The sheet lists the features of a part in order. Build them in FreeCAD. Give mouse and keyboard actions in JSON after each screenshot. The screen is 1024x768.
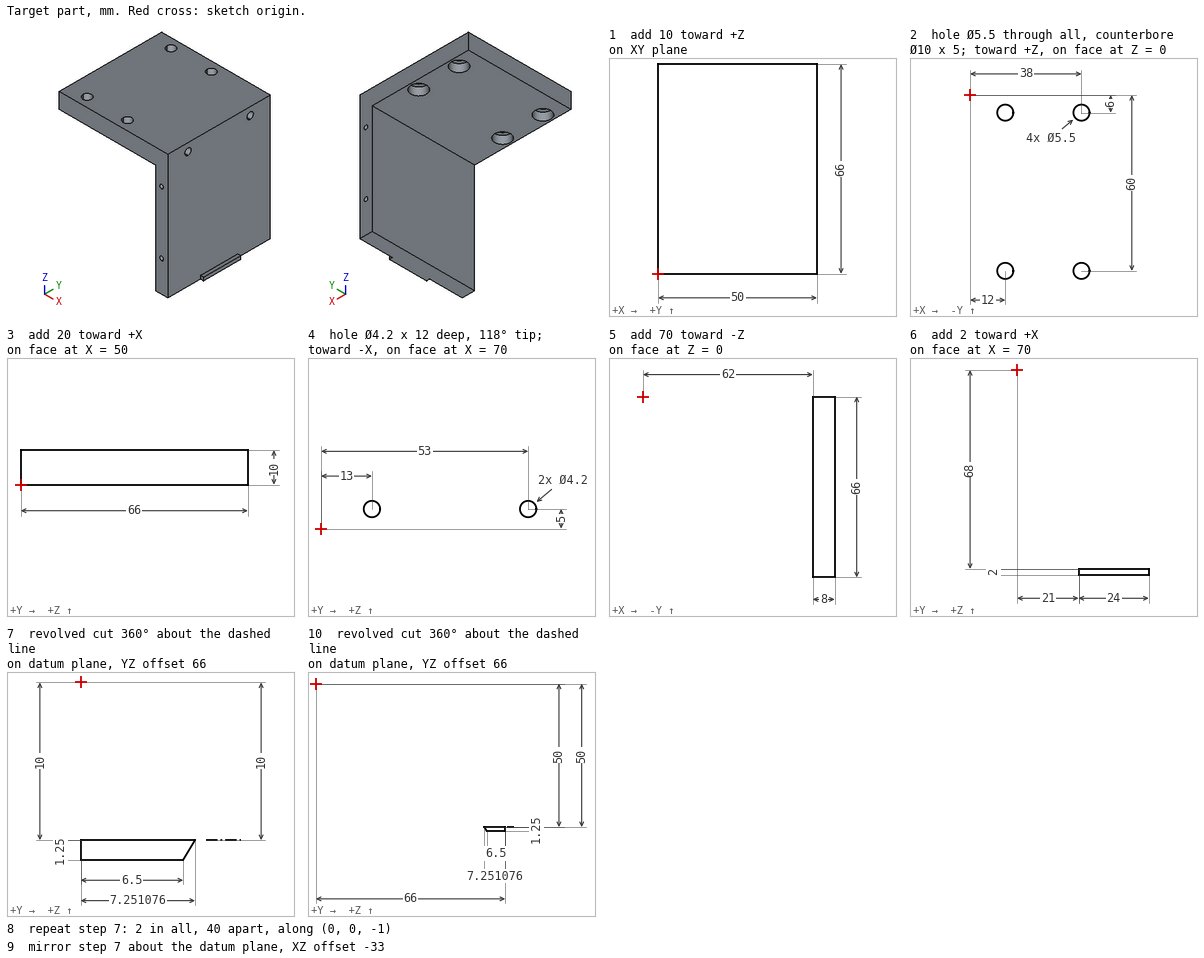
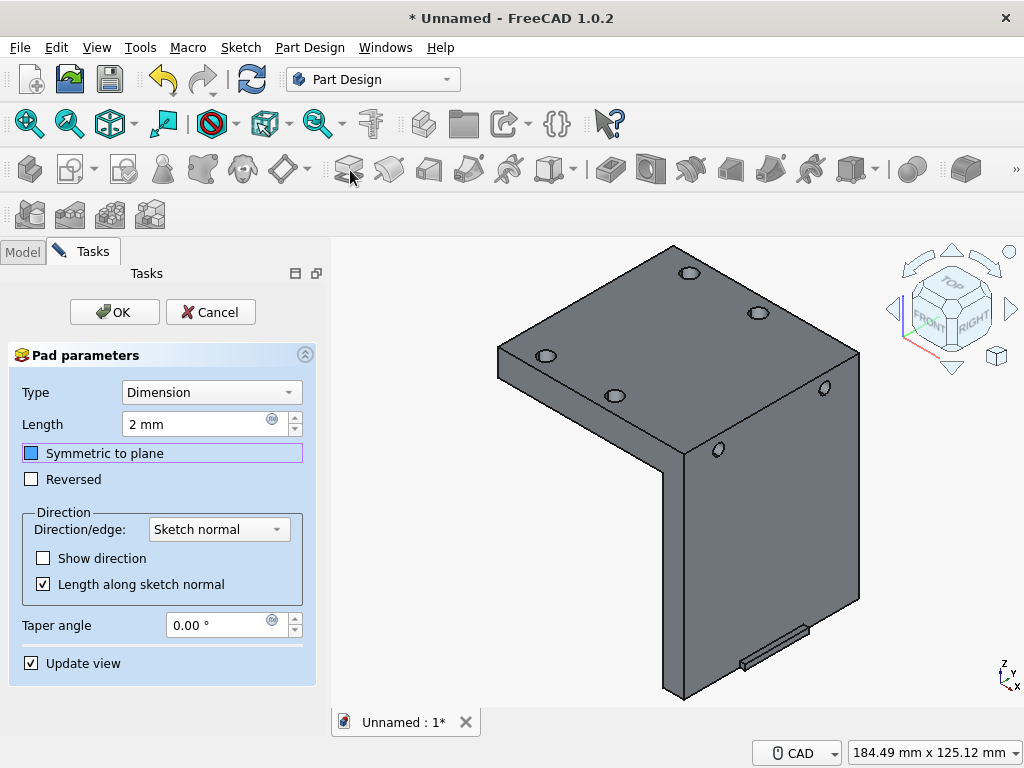
{"action": "left_click", "coordinate": [115, 312]}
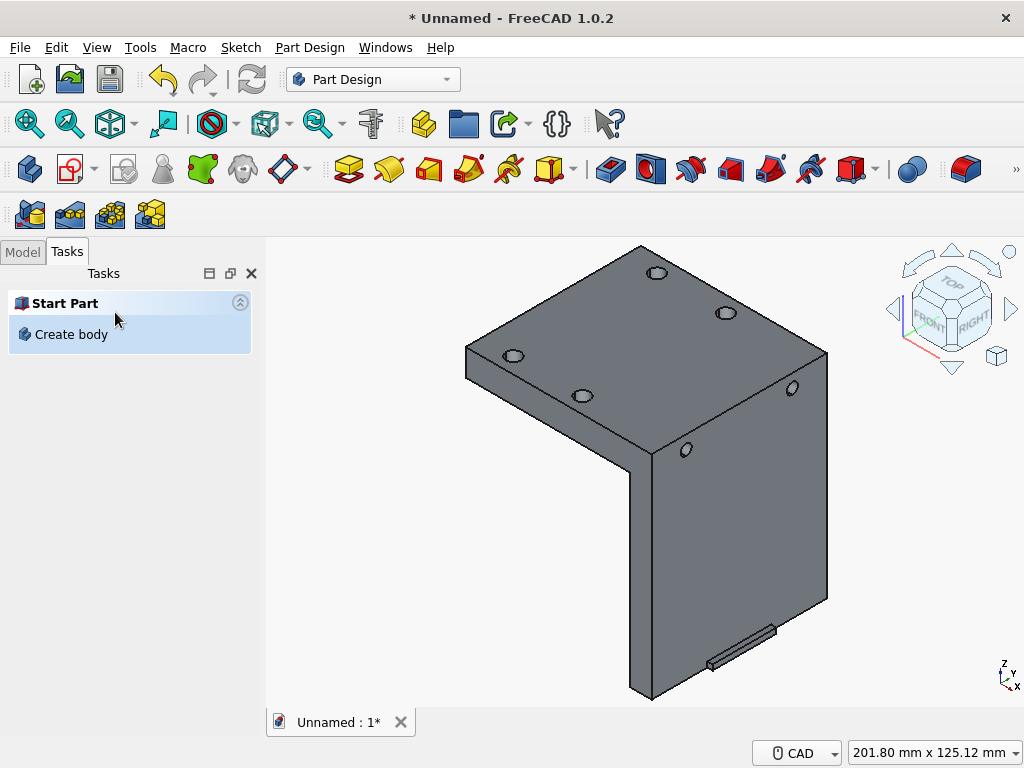
{"action": "left_click", "coordinate": [23, 251]}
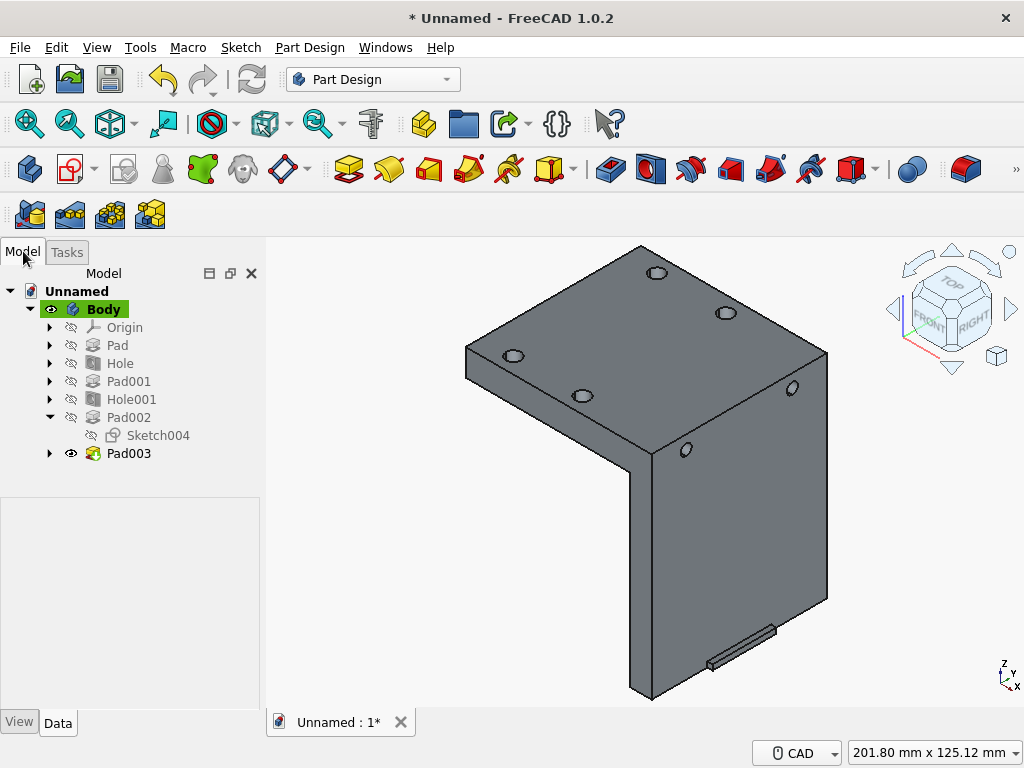
{"action": "left_click", "coordinate": [50, 327]}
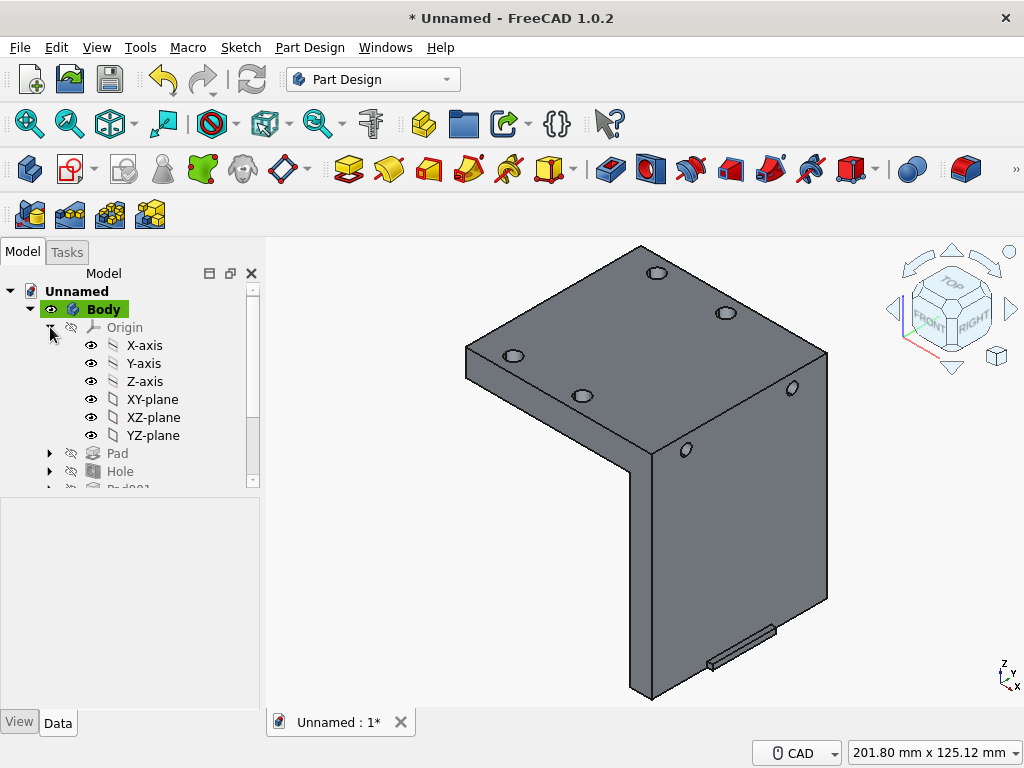
{"action": "left_click", "coordinate": [136, 435]}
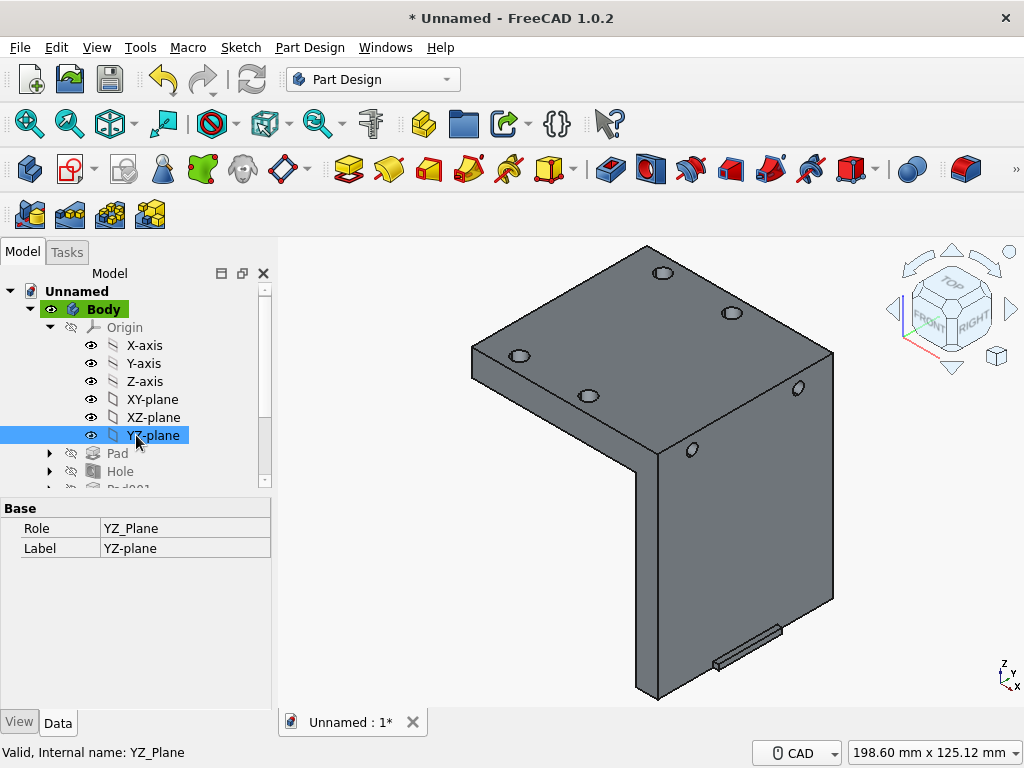
{"action": "left_click", "coordinate": [284, 170]}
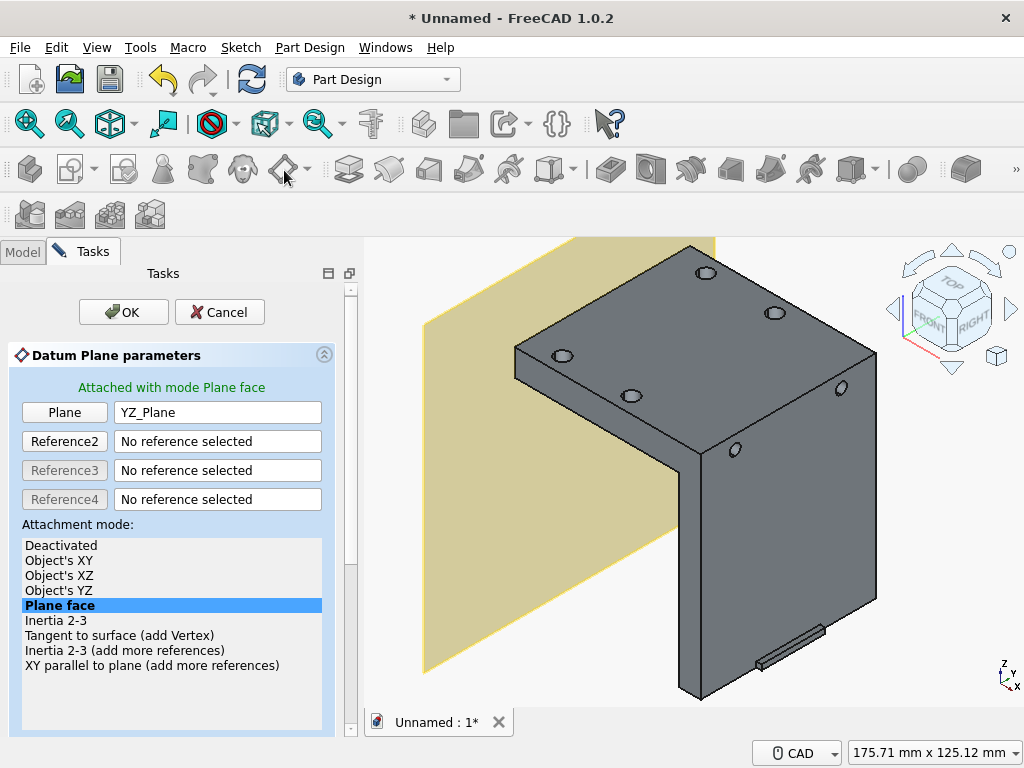
{"action": "scroll", "coordinate": [351, 510], "scroll_direction": "down", "scroll_amount": 3}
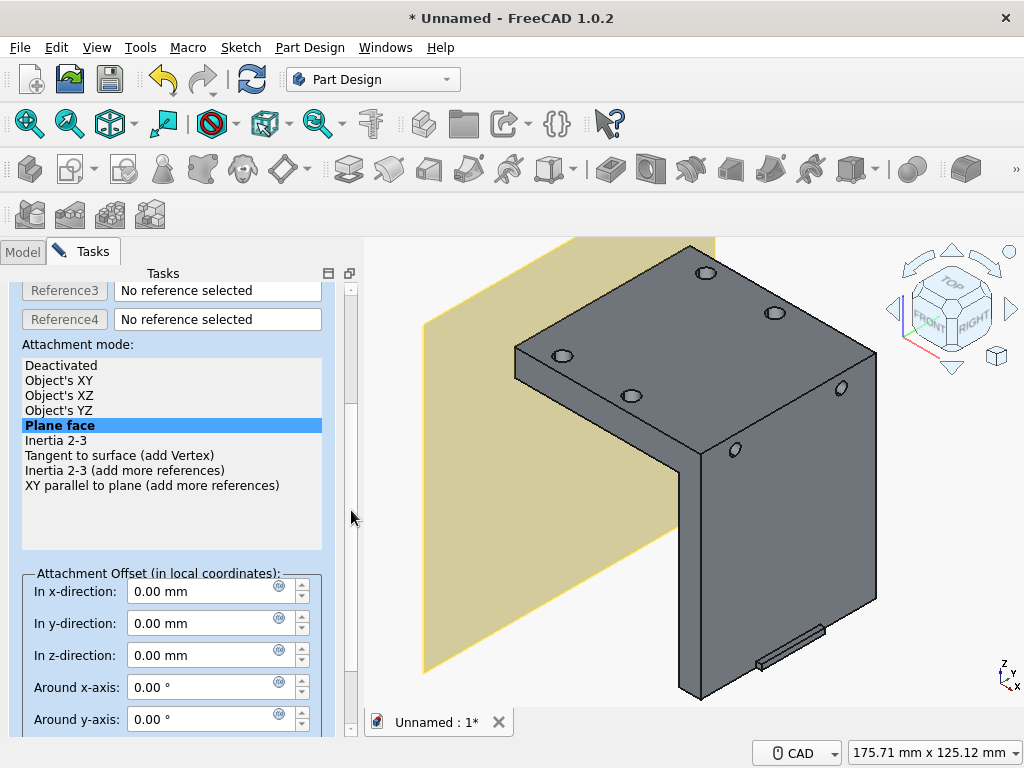
{"action": "triple_click", "coordinate": [210, 655]}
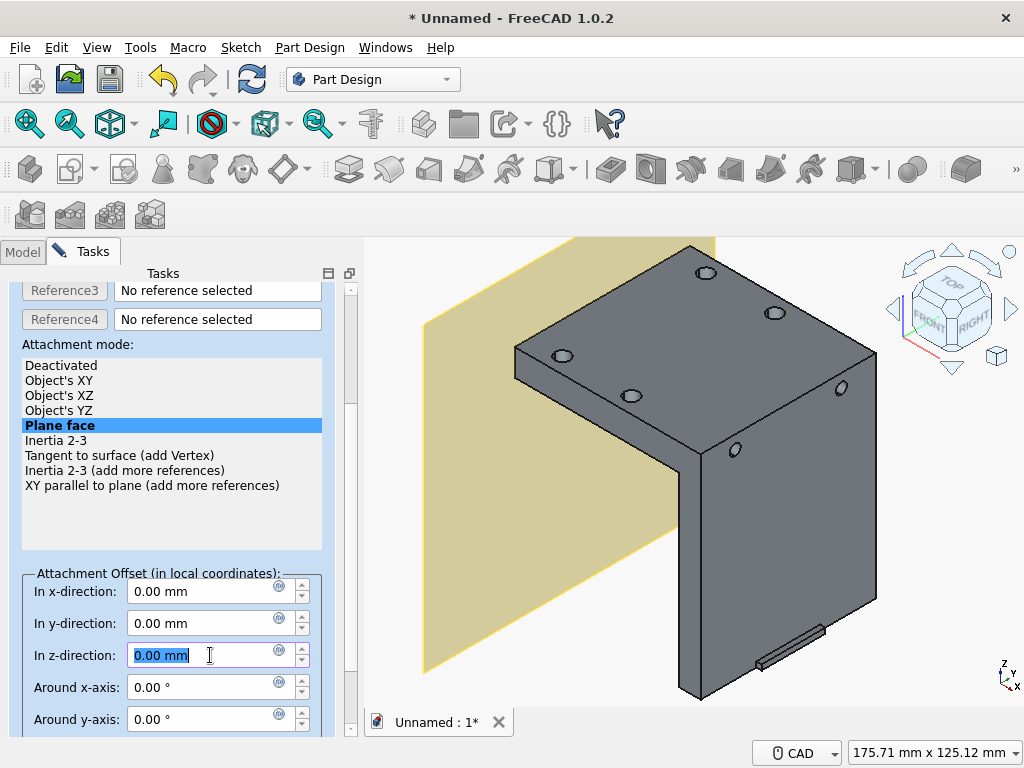
{"action": "type", "text": "66"}
{"action": "key", "text": "Tab"}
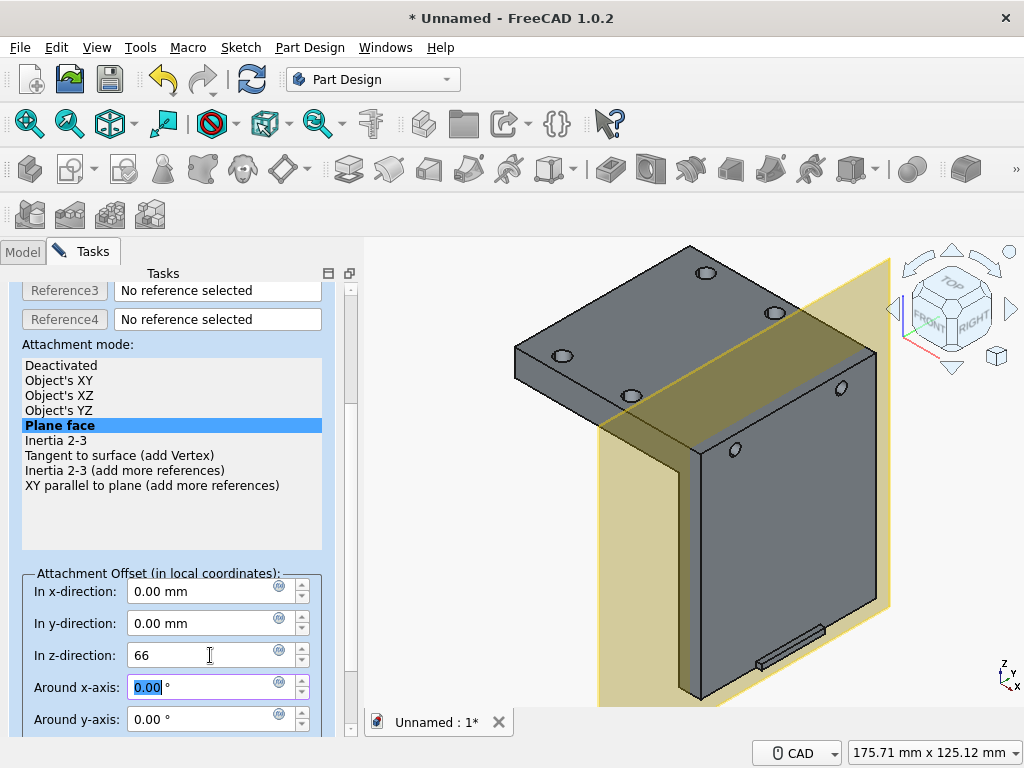
{"action": "scroll", "coordinate": [351, 510], "scroll_direction": "up", "scroll_amount": 4}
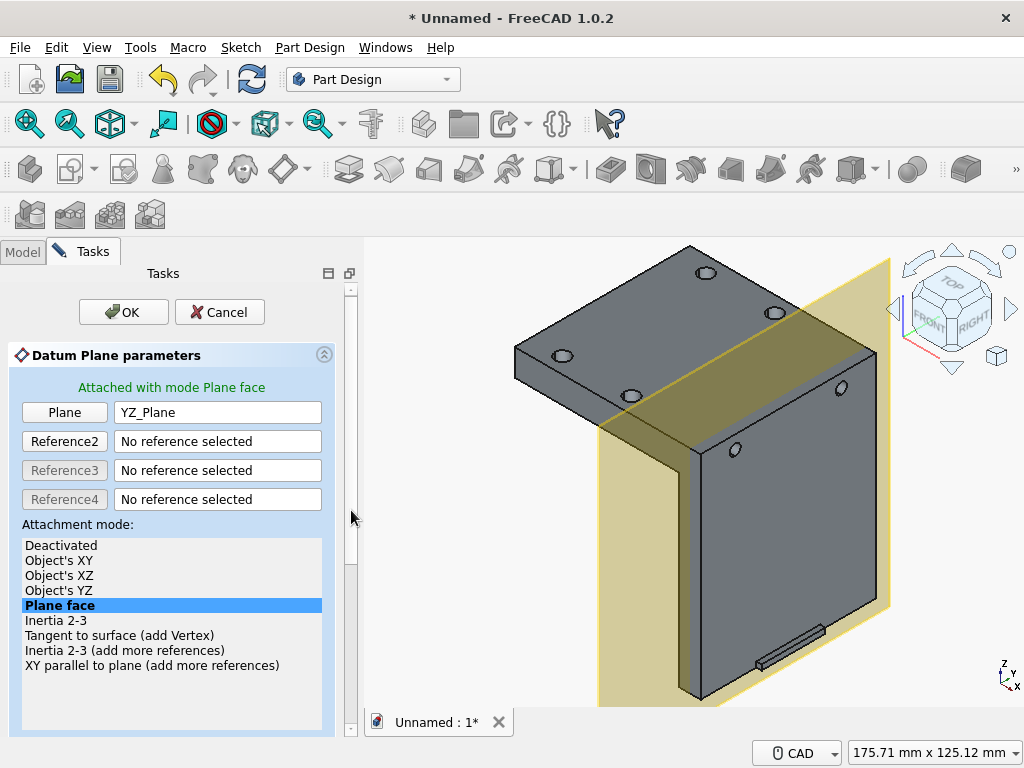
{"action": "left_click", "coordinate": [124, 312]}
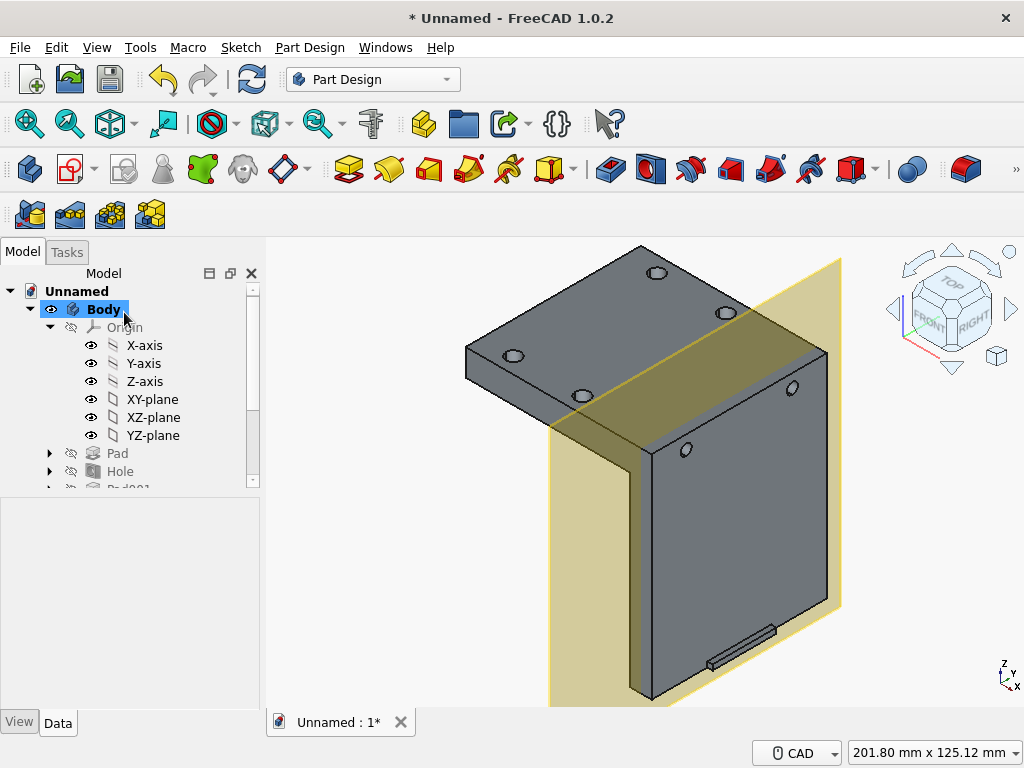
{"action": "scroll", "coordinate": [100, 377], "scroll_direction": "down", "scroll_amount": 3}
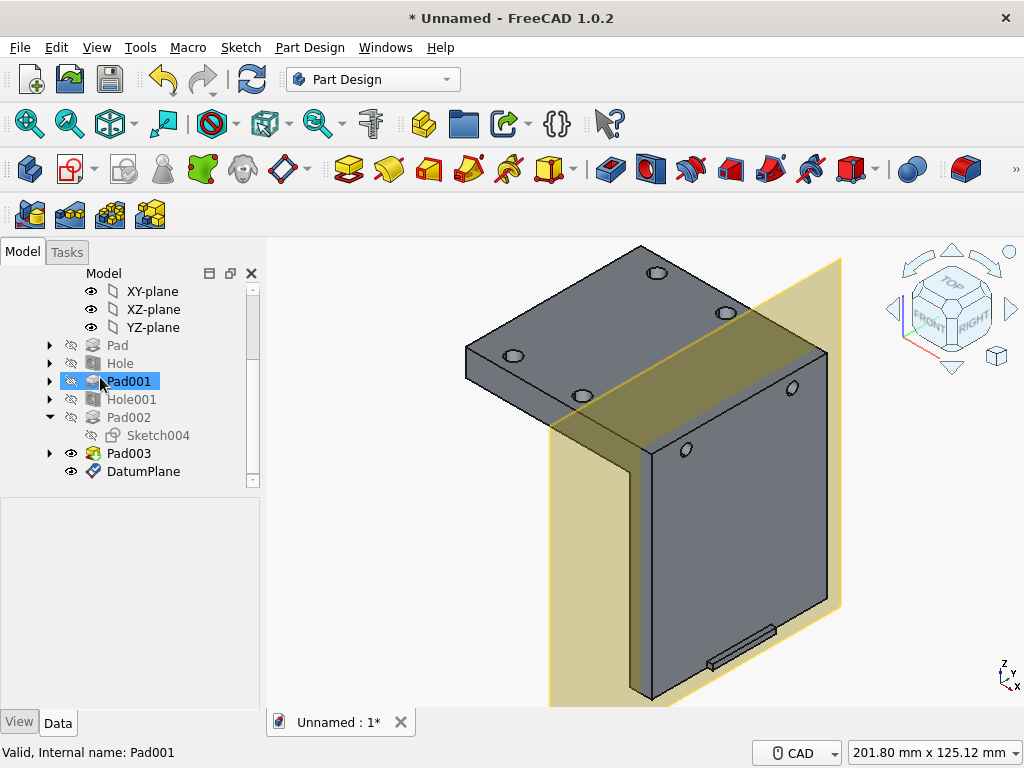
{"action": "left_click", "coordinate": [116, 471]}